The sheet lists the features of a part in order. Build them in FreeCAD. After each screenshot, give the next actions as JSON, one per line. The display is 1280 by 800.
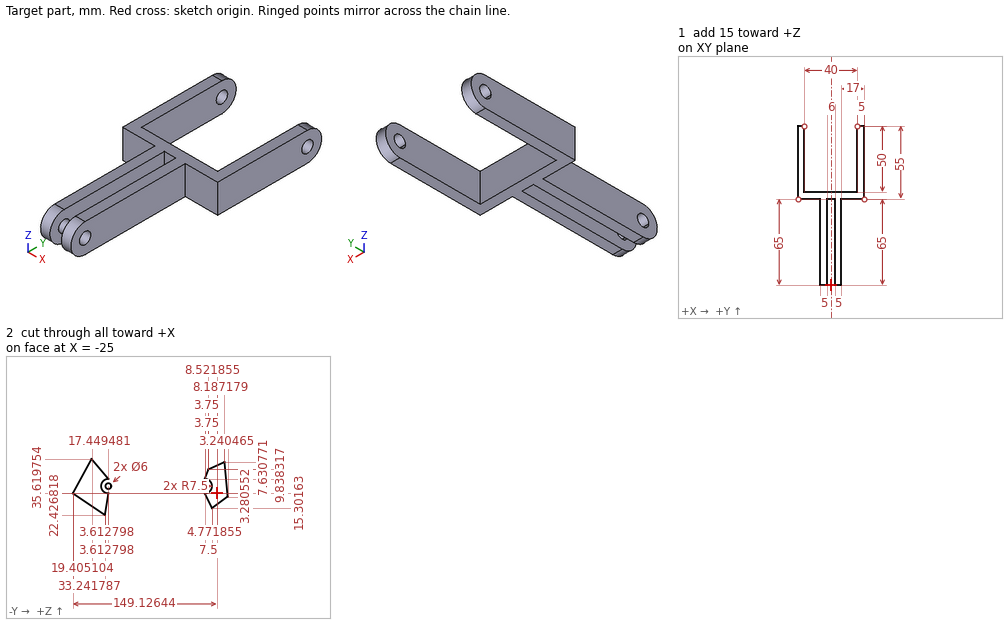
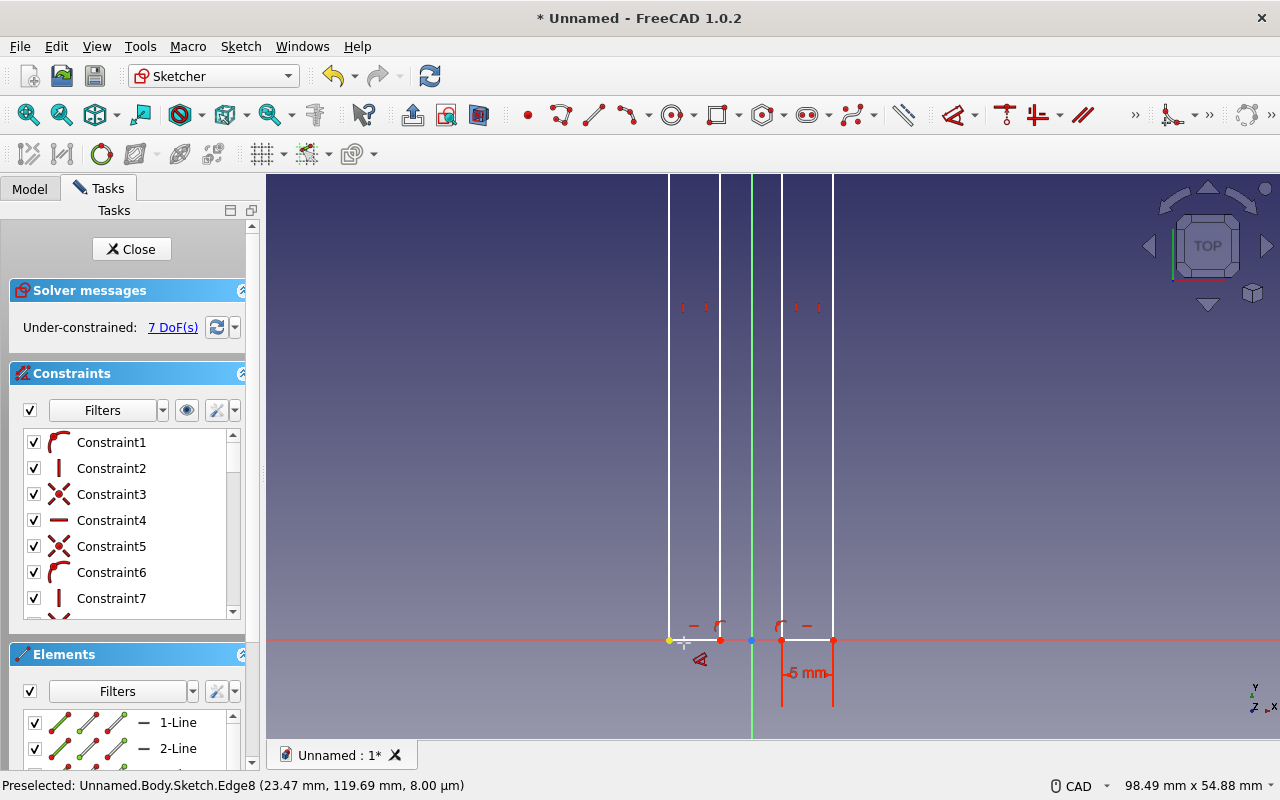
{"action": "left_click", "coordinate": [685, 640]}
{"action": "left_click", "coordinate": [695, 674]}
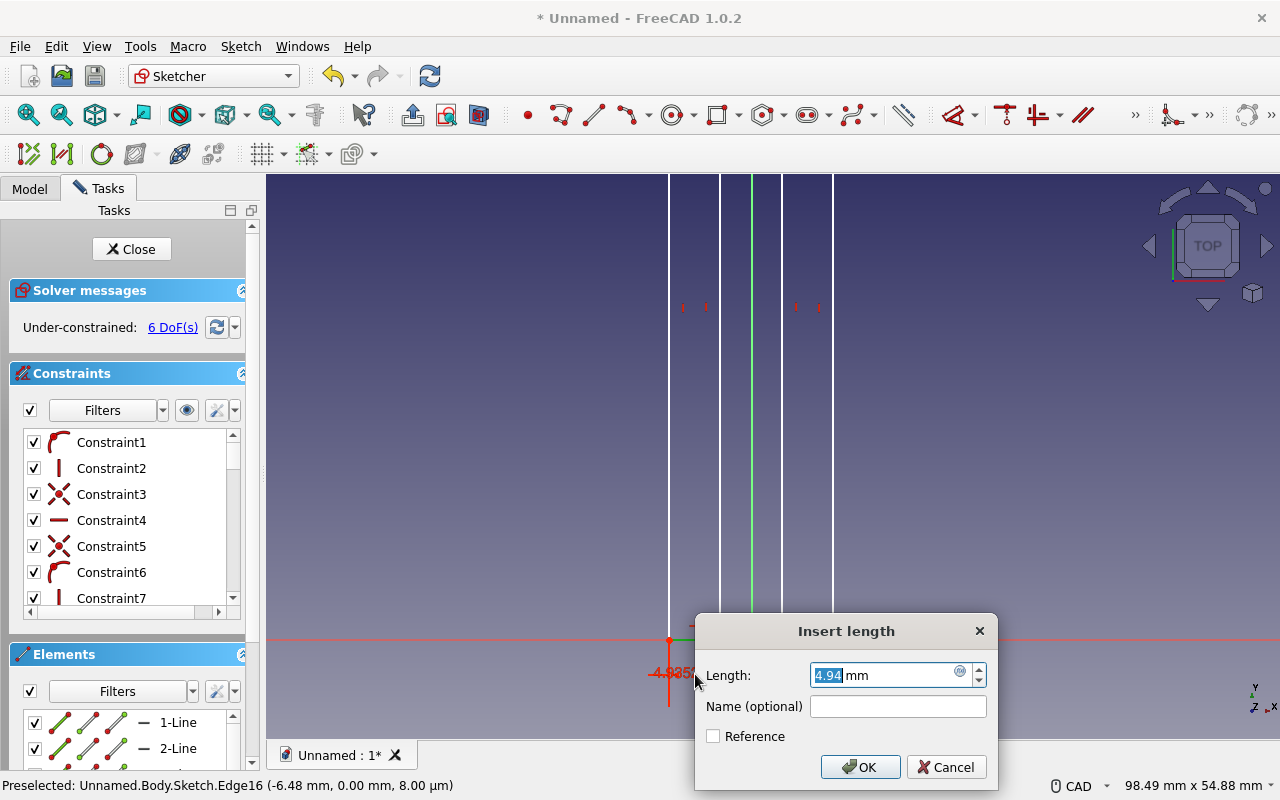
{"action": "type", "text": "5"}
{"action": "key", "text": "Return"}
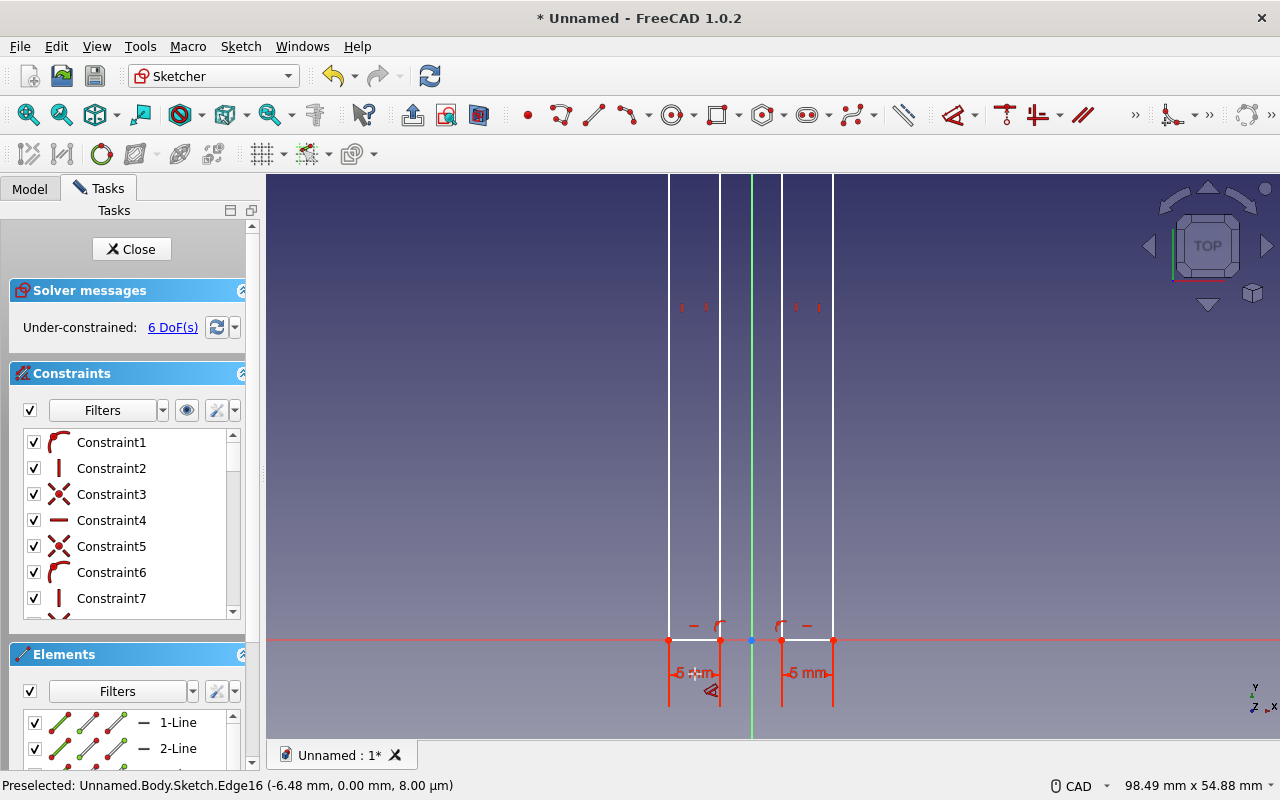
{"action": "left_click", "coordinate": [720, 440]}
{"action": "left_click", "coordinate": [686, 421]}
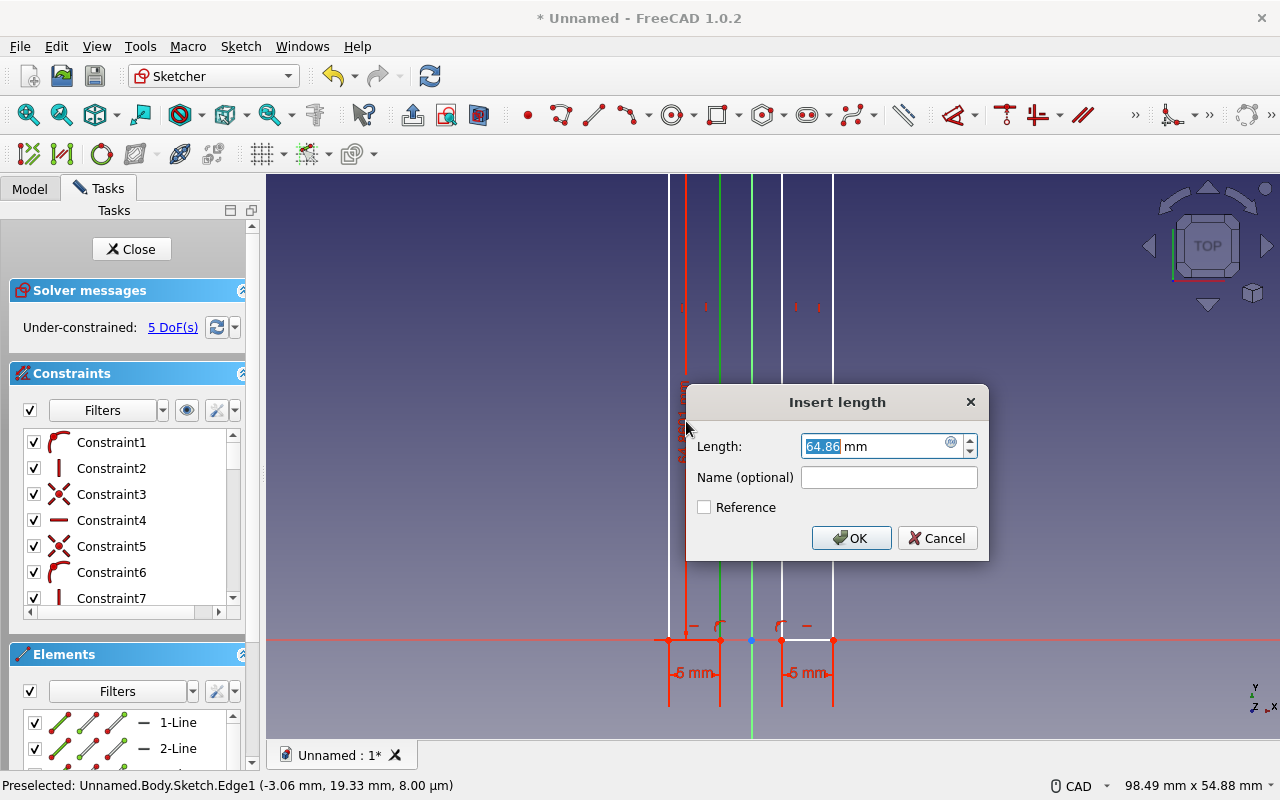
{"action": "type", "text": "65"}
{"action": "key", "text": "Return"}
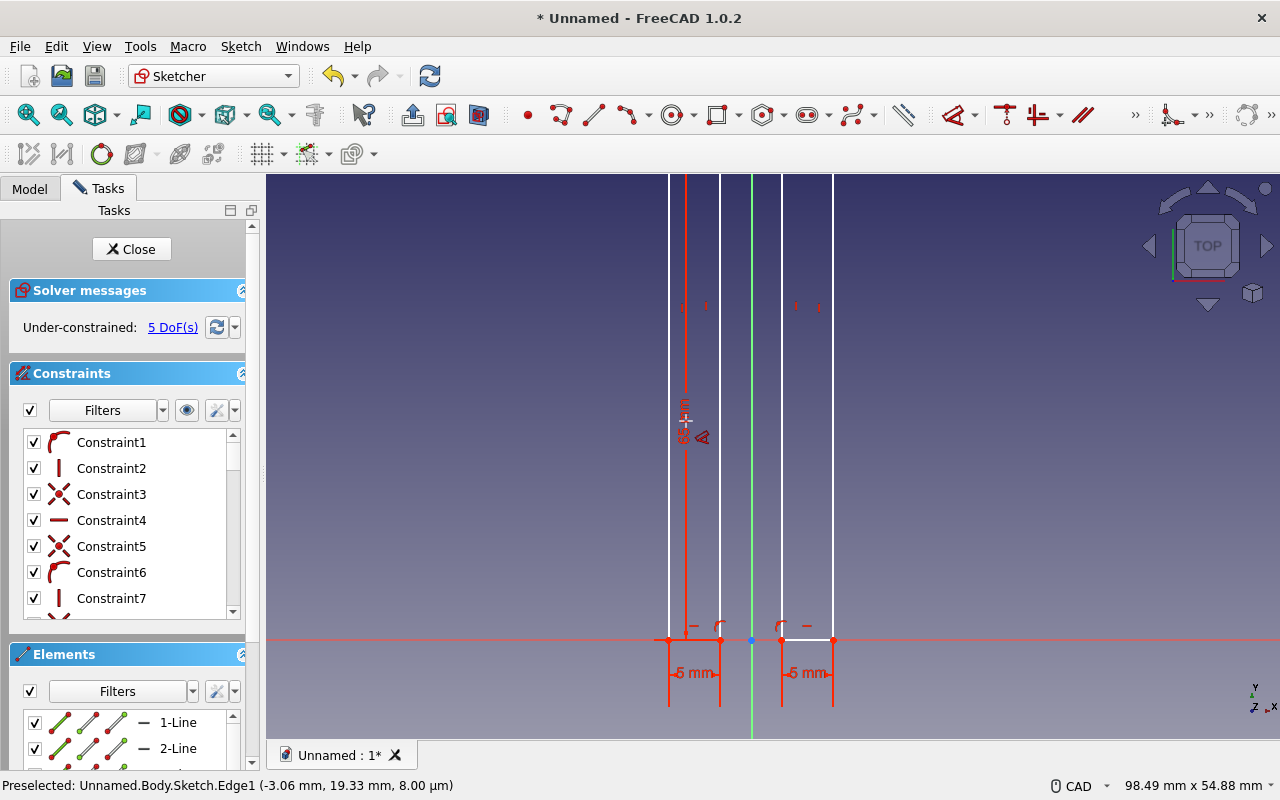
{"action": "scroll", "coordinate": [684, 644], "scroll_direction": "down", "scroll_amount": 6}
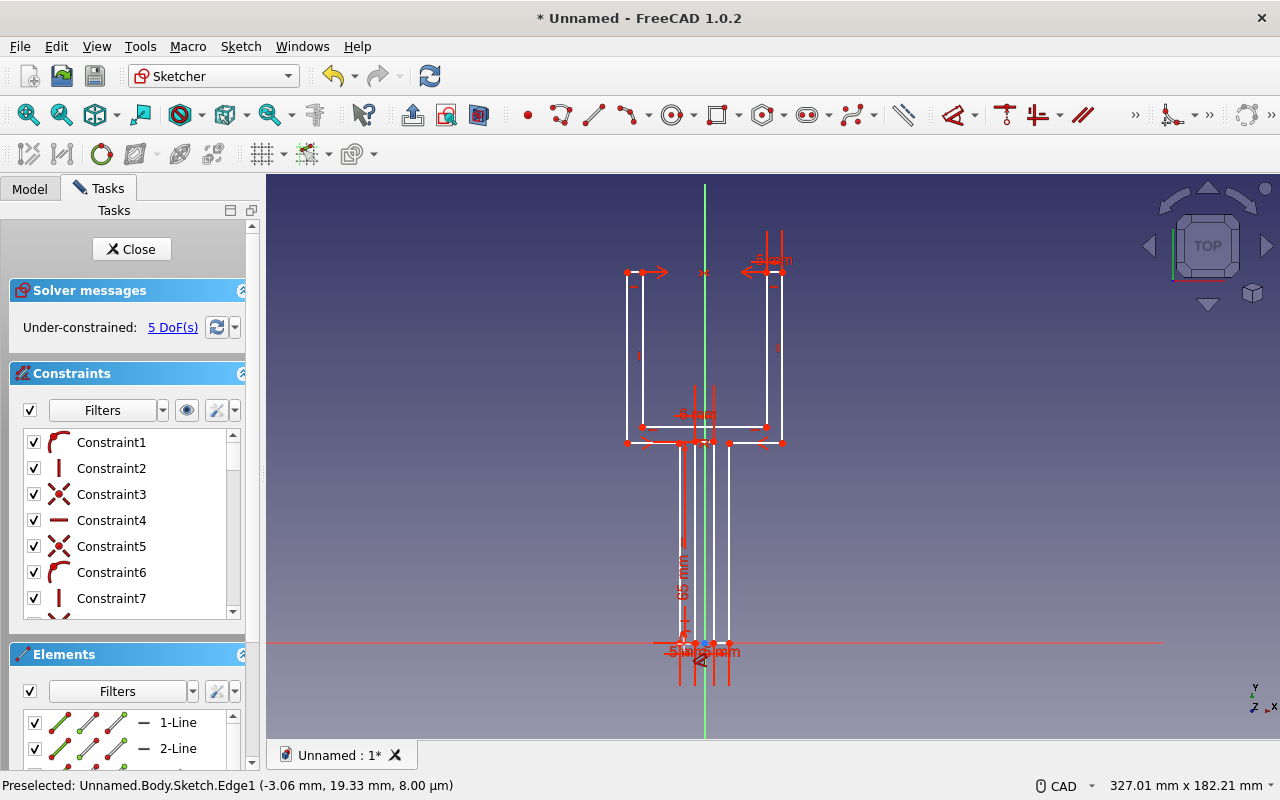
{"action": "left_click", "coordinate": [729, 583]}
{"action": "left_click", "coordinate": [763, 543]}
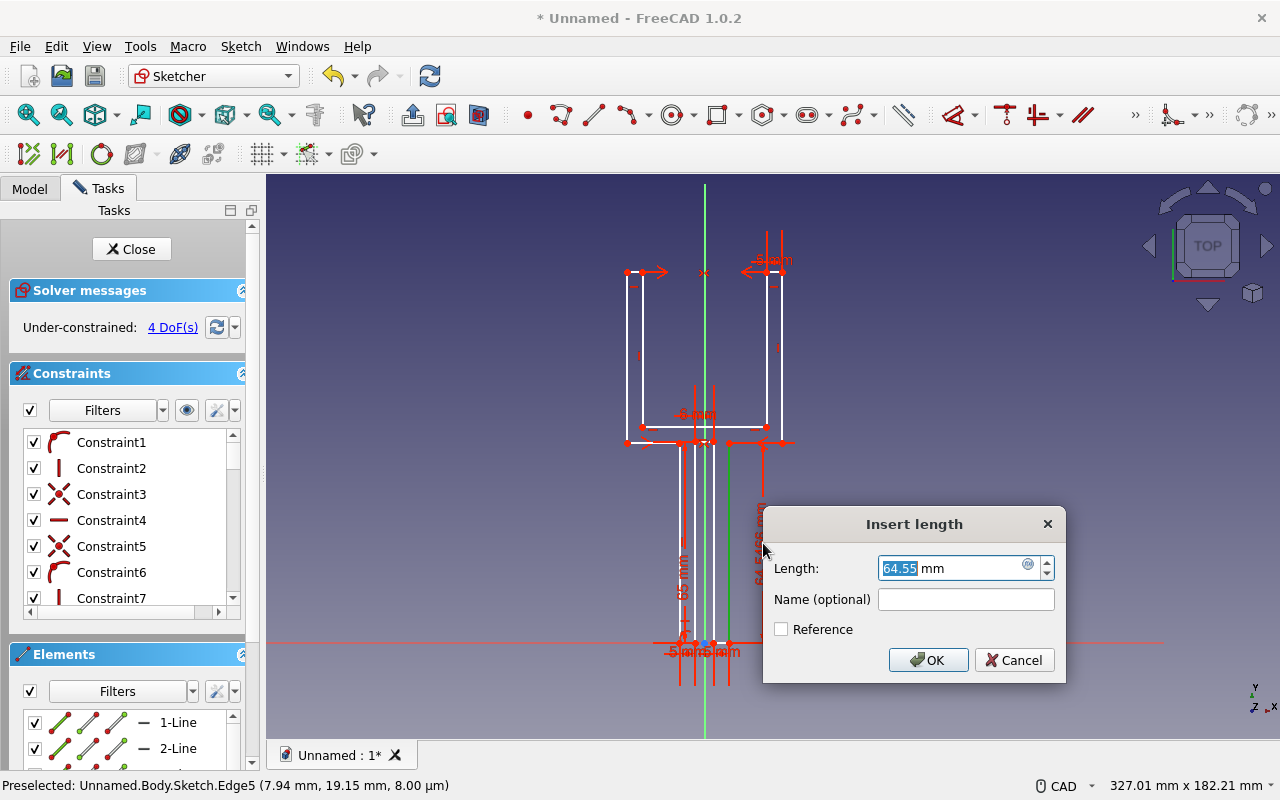
{"action": "type", "text": "65"}
{"action": "key", "text": "Return"}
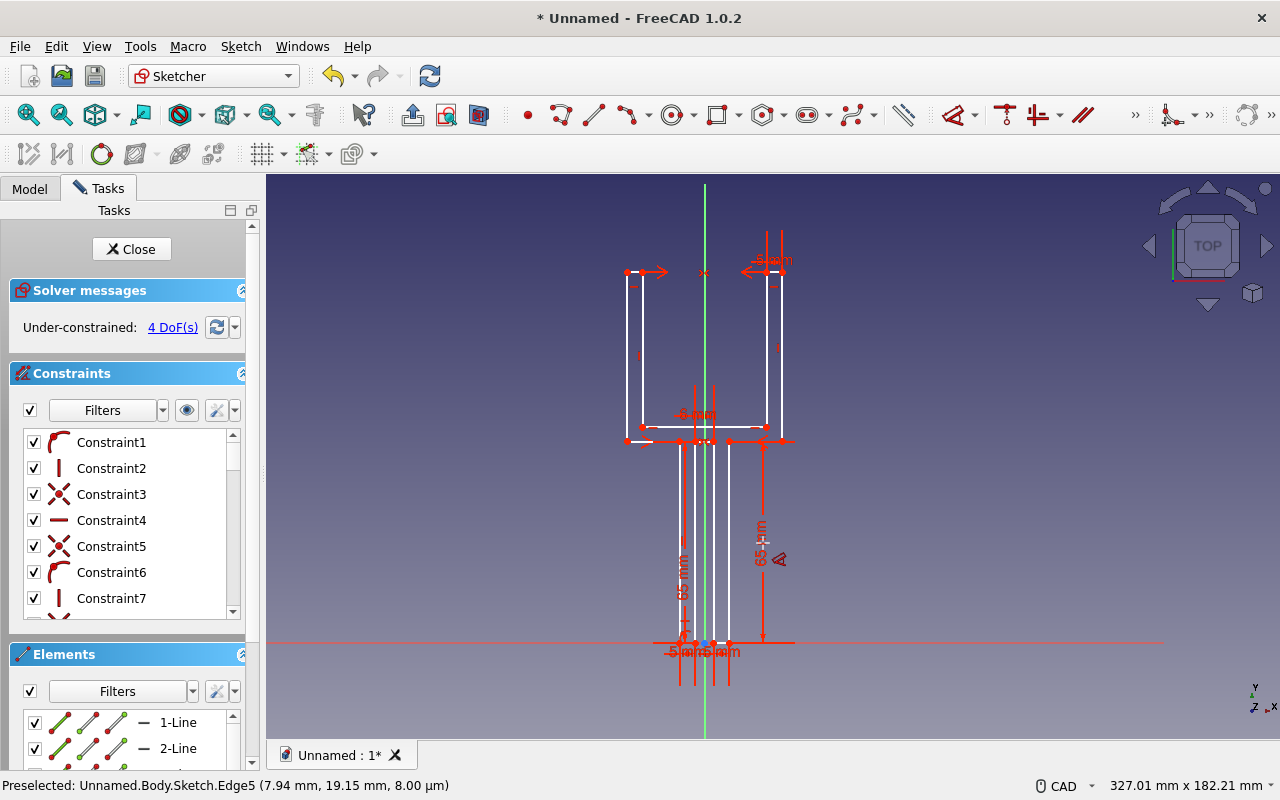
{"action": "left_click", "coordinate": [745, 442]}
{"action": "left_click", "coordinate": [756, 476]}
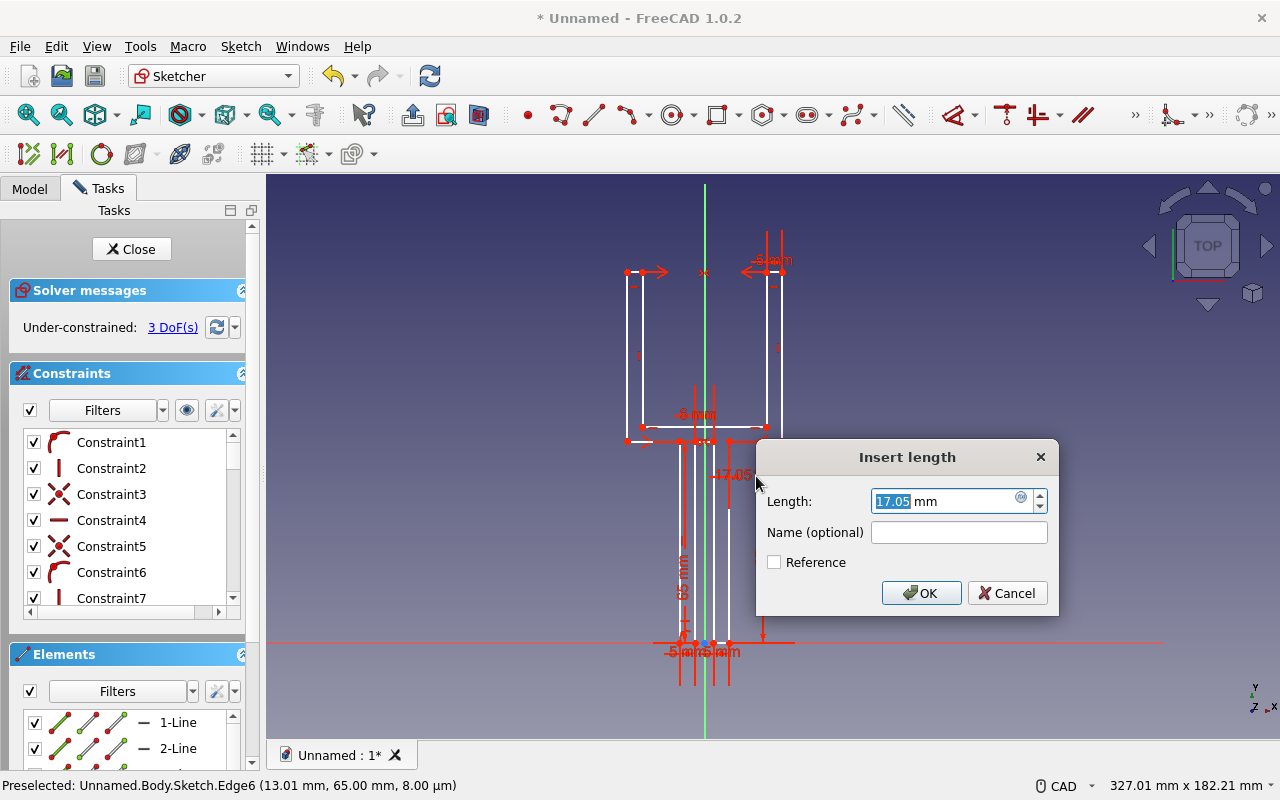
{"action": "type", "text": "17"}
{"action": "key", "text": "Return"}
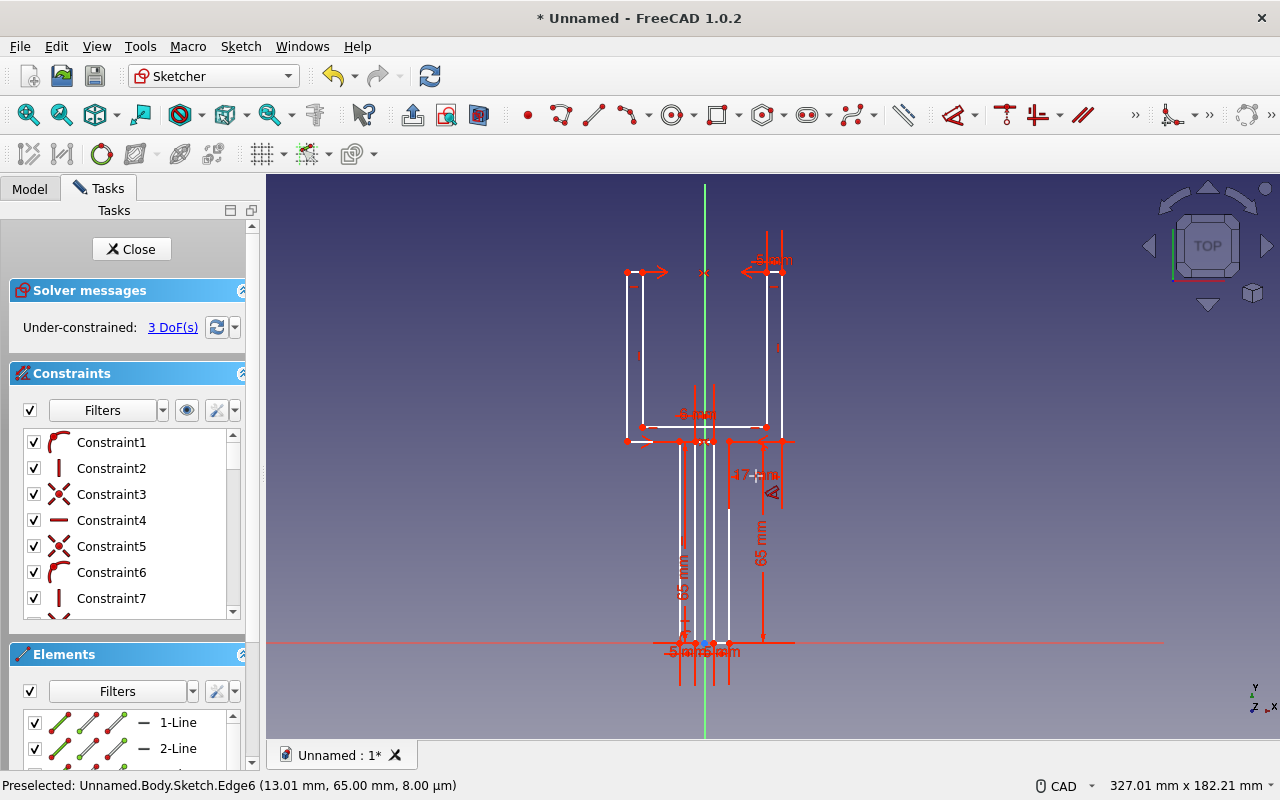
{"action": "left_click", "coordinate": [782, 391]}
{"action": "left_click", "coordinate": [816, 357]}